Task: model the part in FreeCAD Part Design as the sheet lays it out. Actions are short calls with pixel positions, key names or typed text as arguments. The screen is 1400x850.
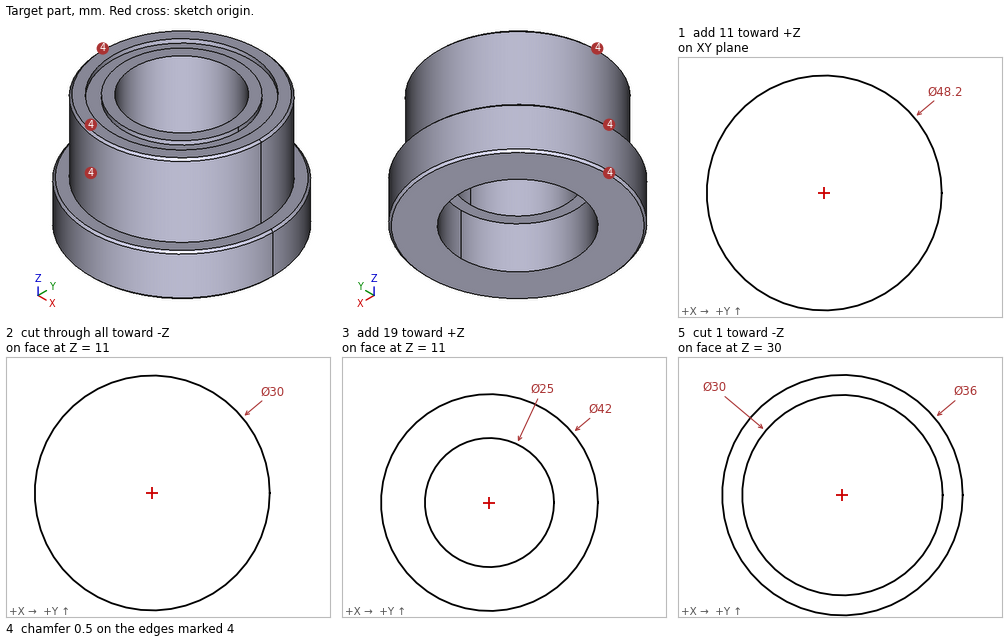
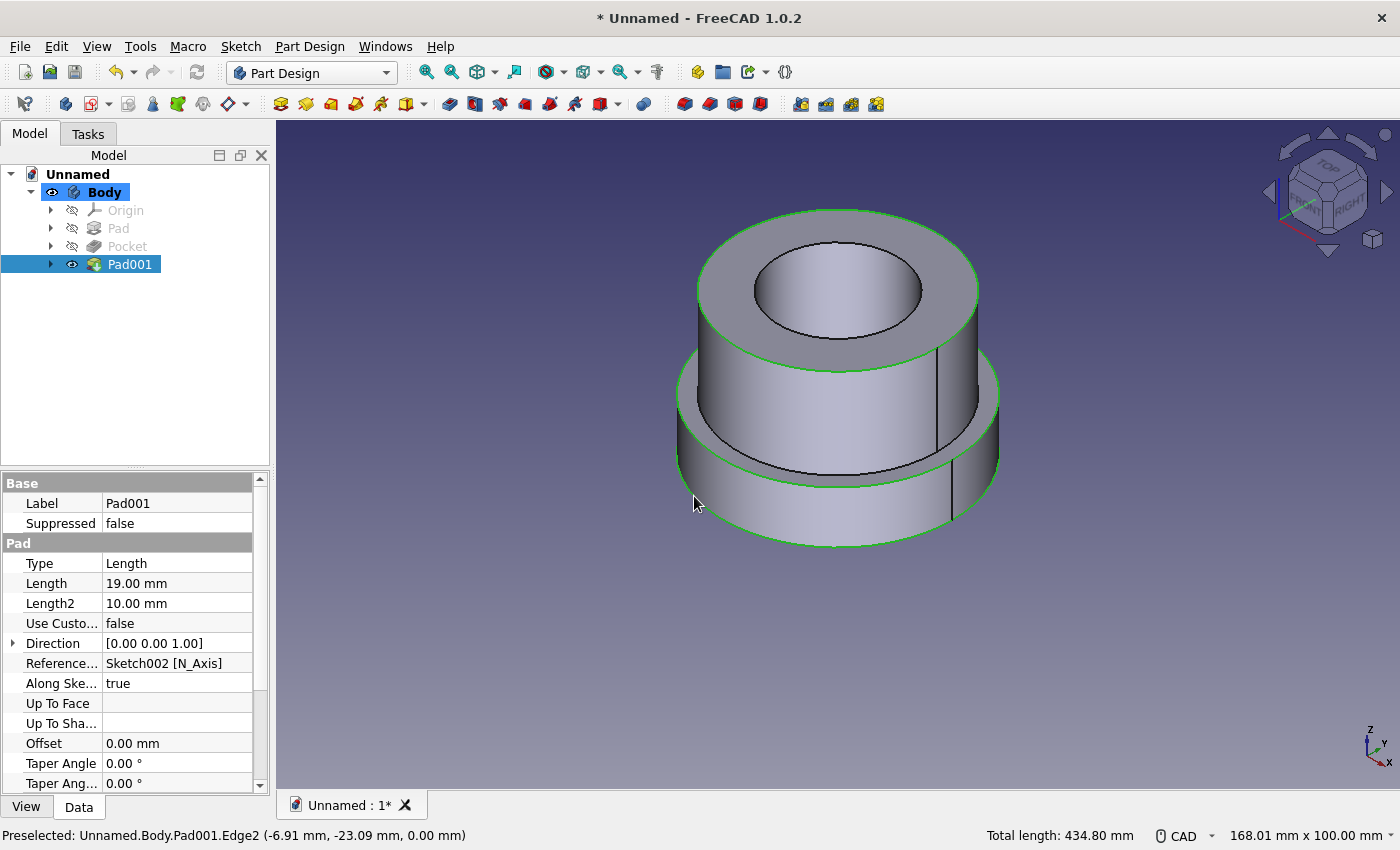
click(710, 104)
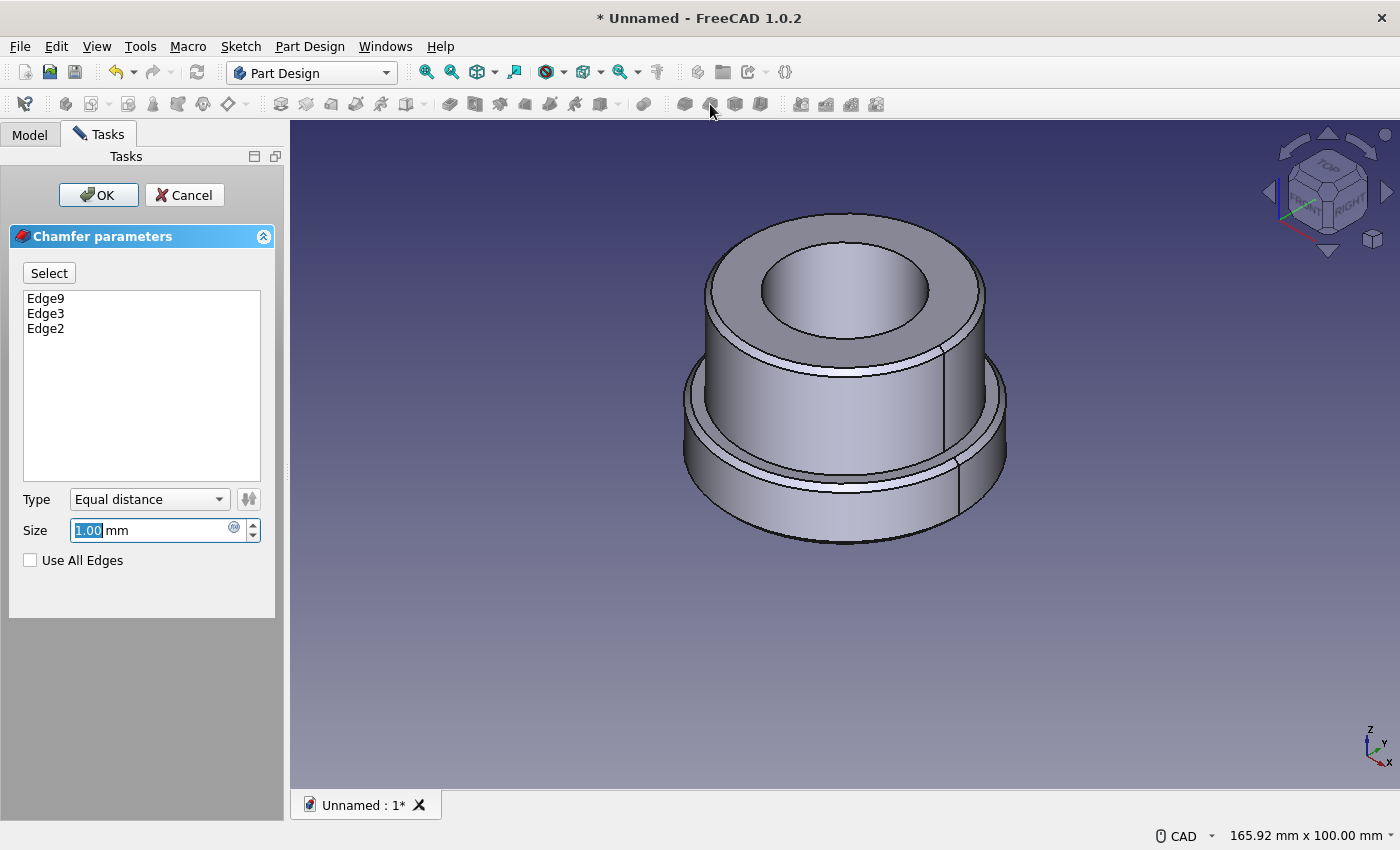
text(0.5)
key(Tab)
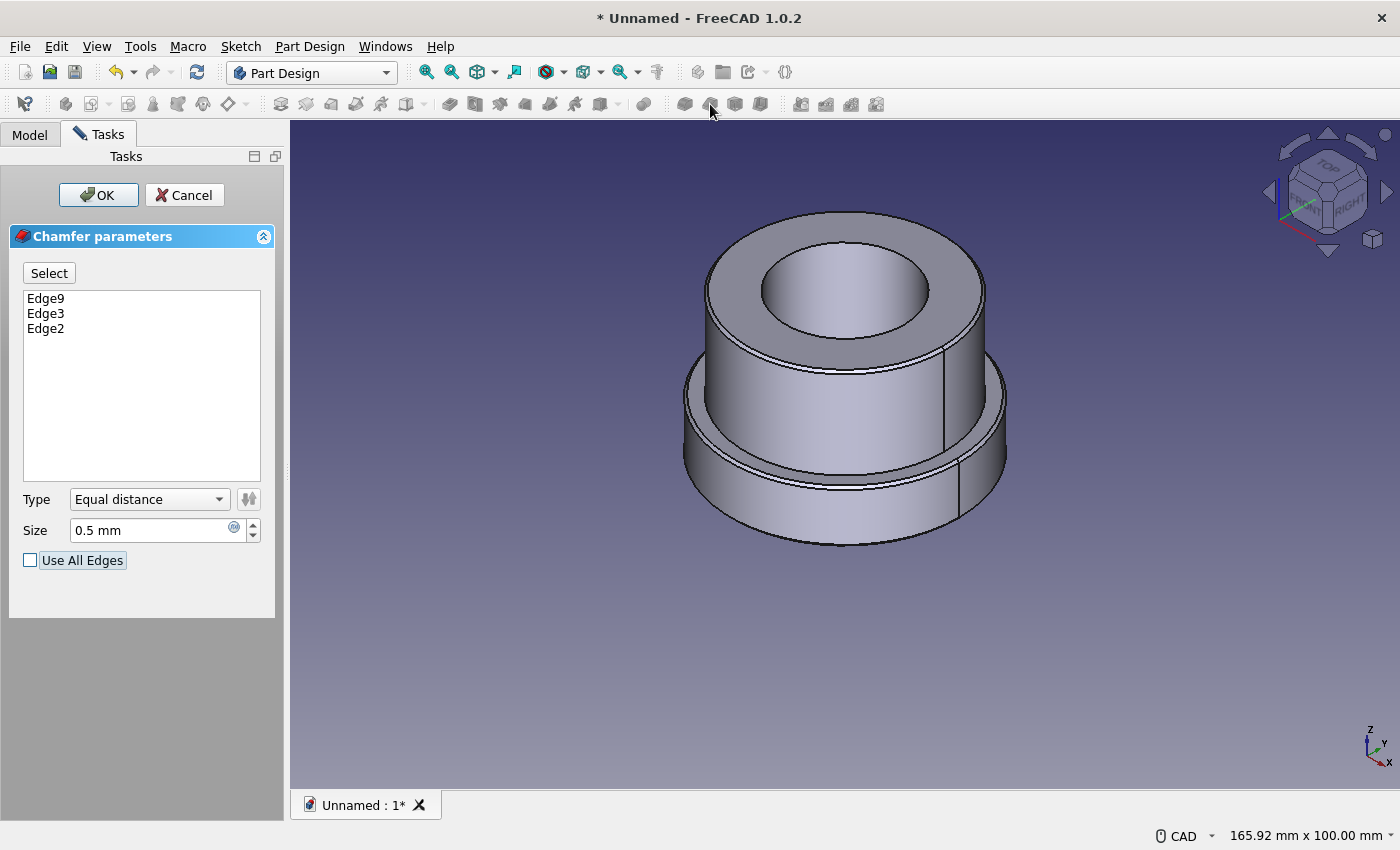
click(99, 195)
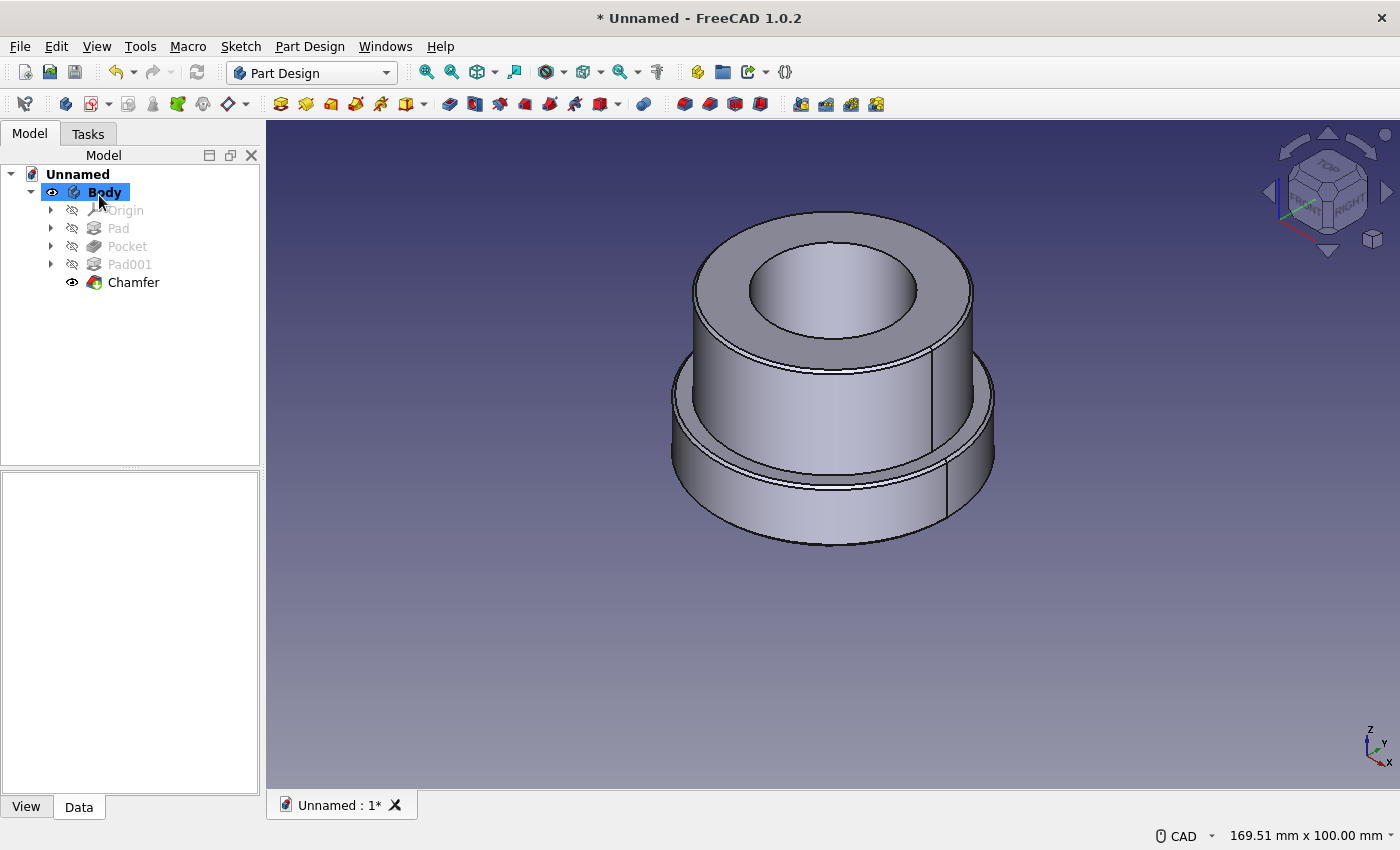
click(722, 290)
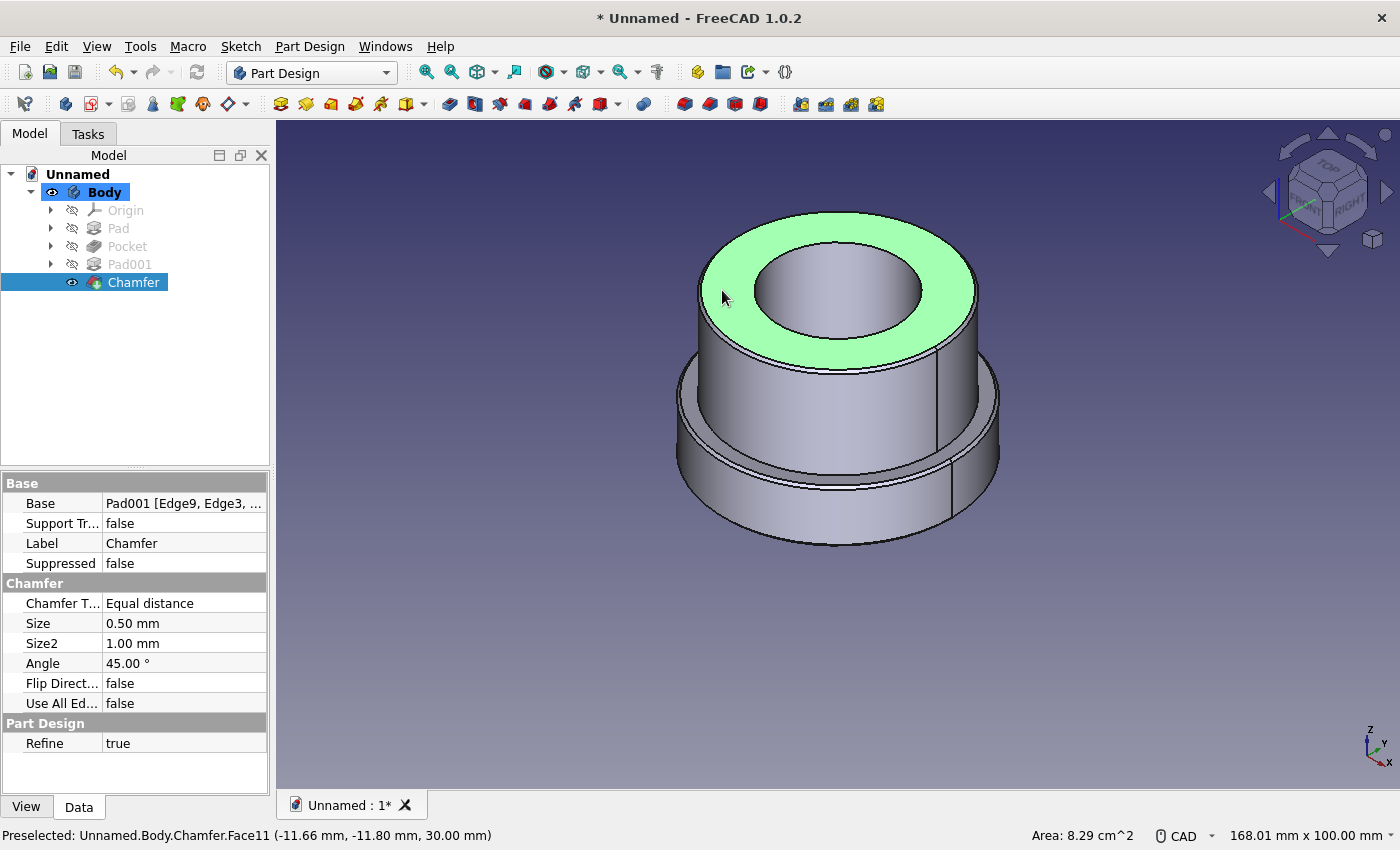
click(90, 104)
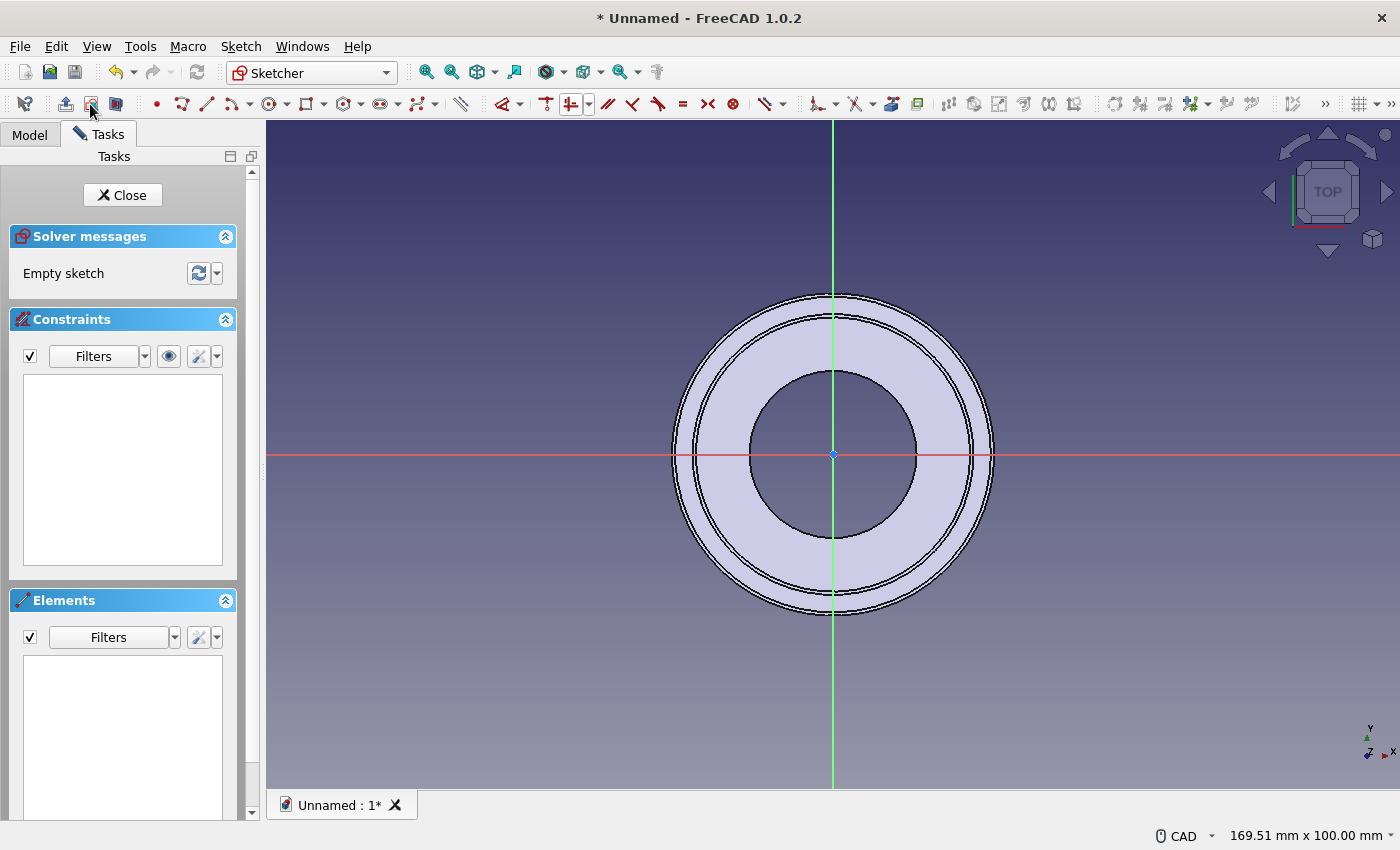
scroll(916, 454, up, 3)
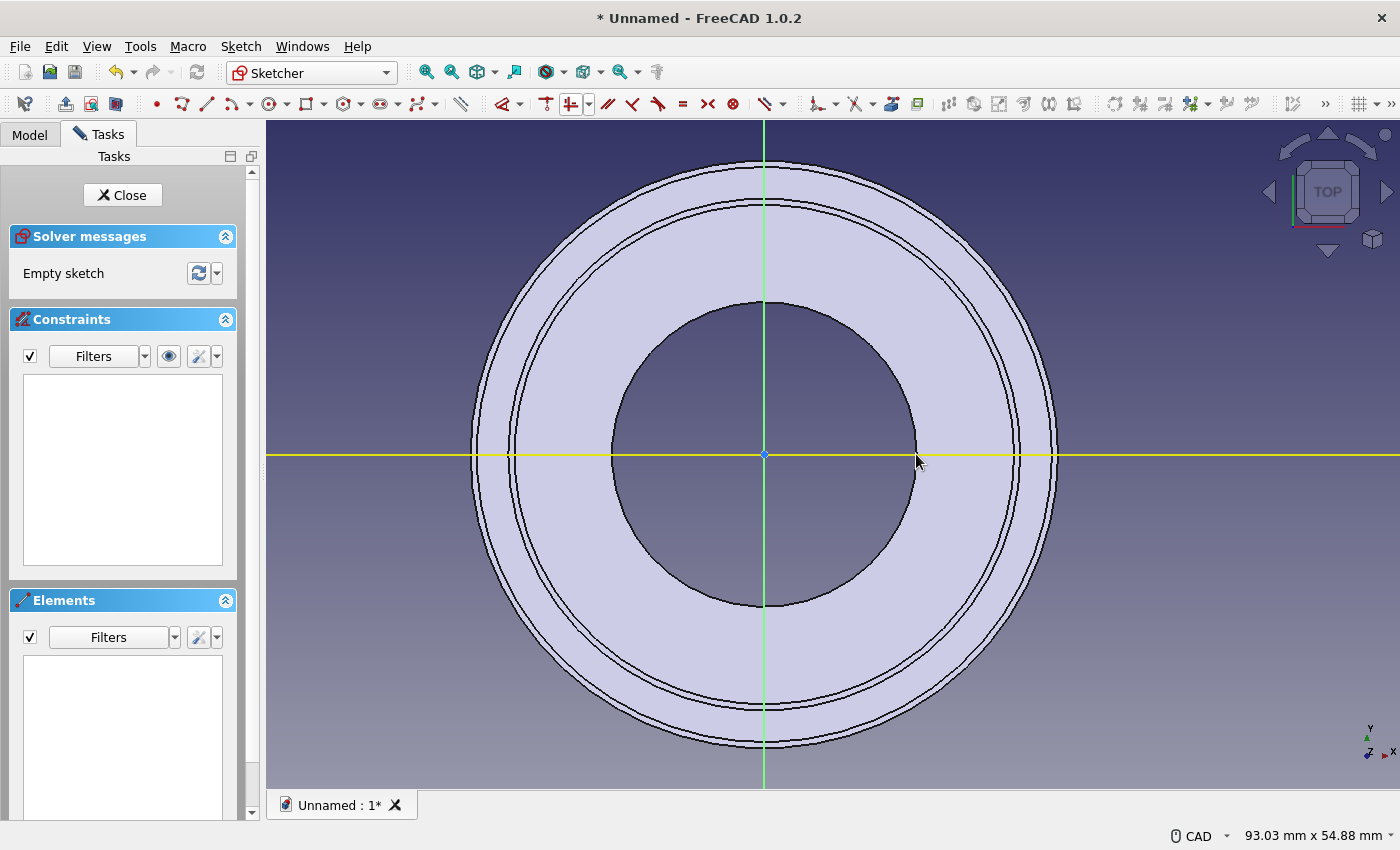
key(g)
key(c)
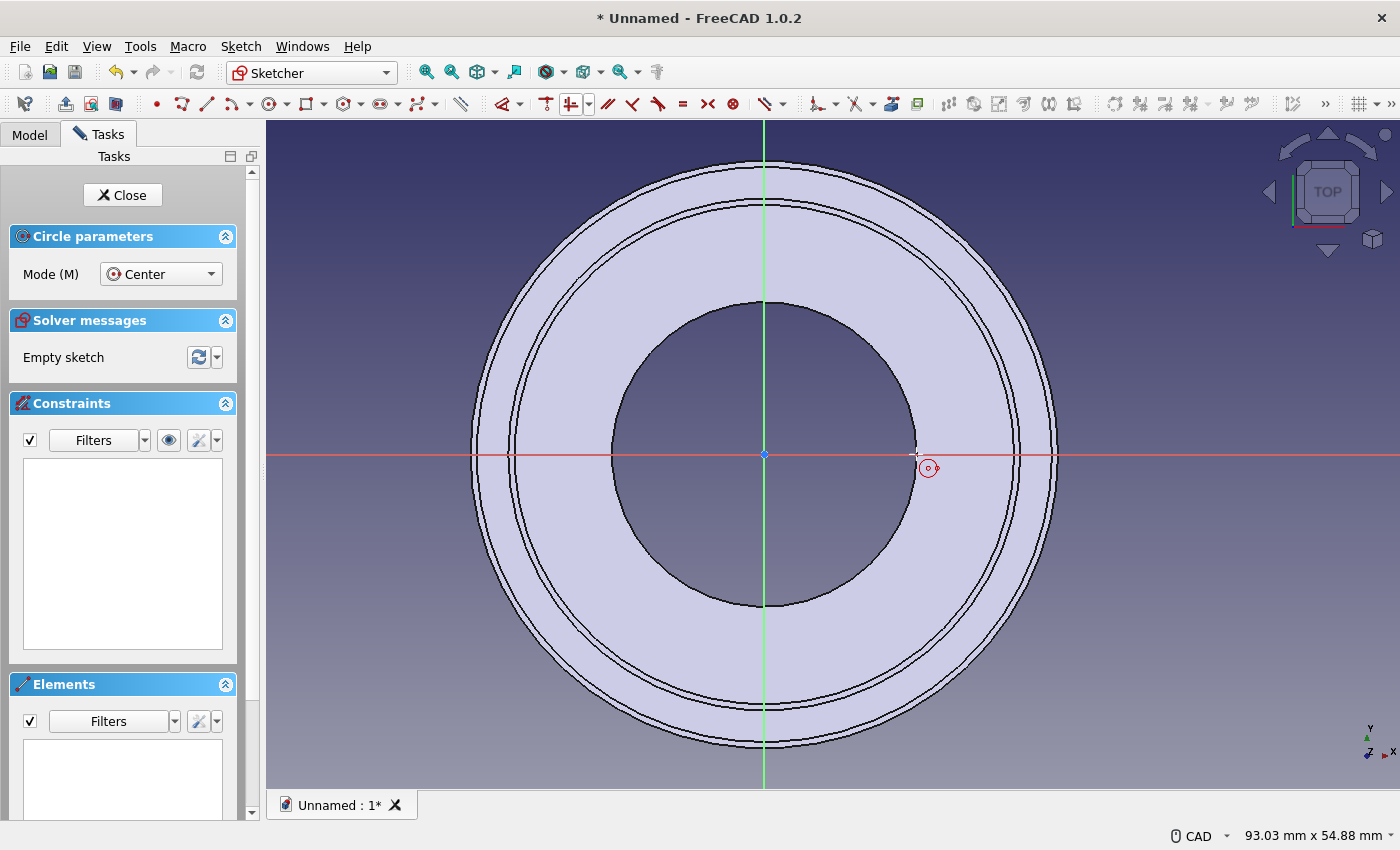
click(764, 454)
click(919, 299)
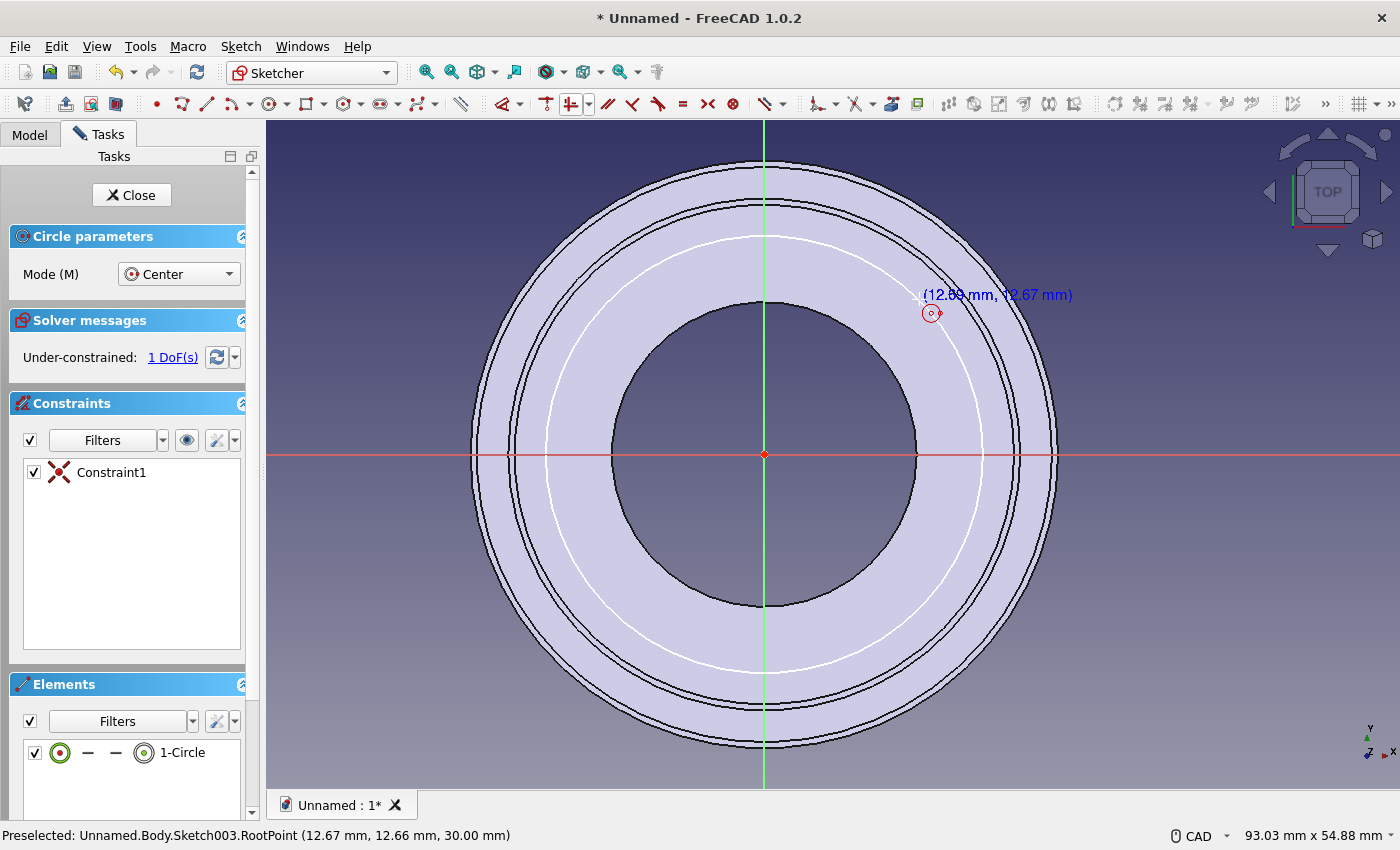
click(764, 454)
click(894, 325)
key(Escape)